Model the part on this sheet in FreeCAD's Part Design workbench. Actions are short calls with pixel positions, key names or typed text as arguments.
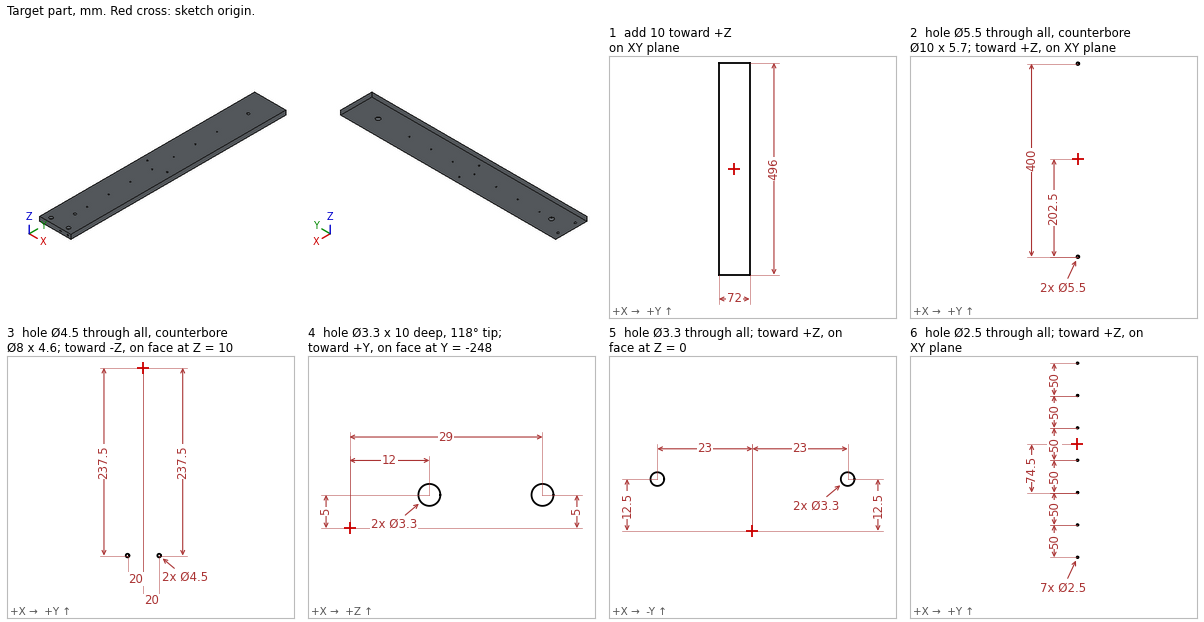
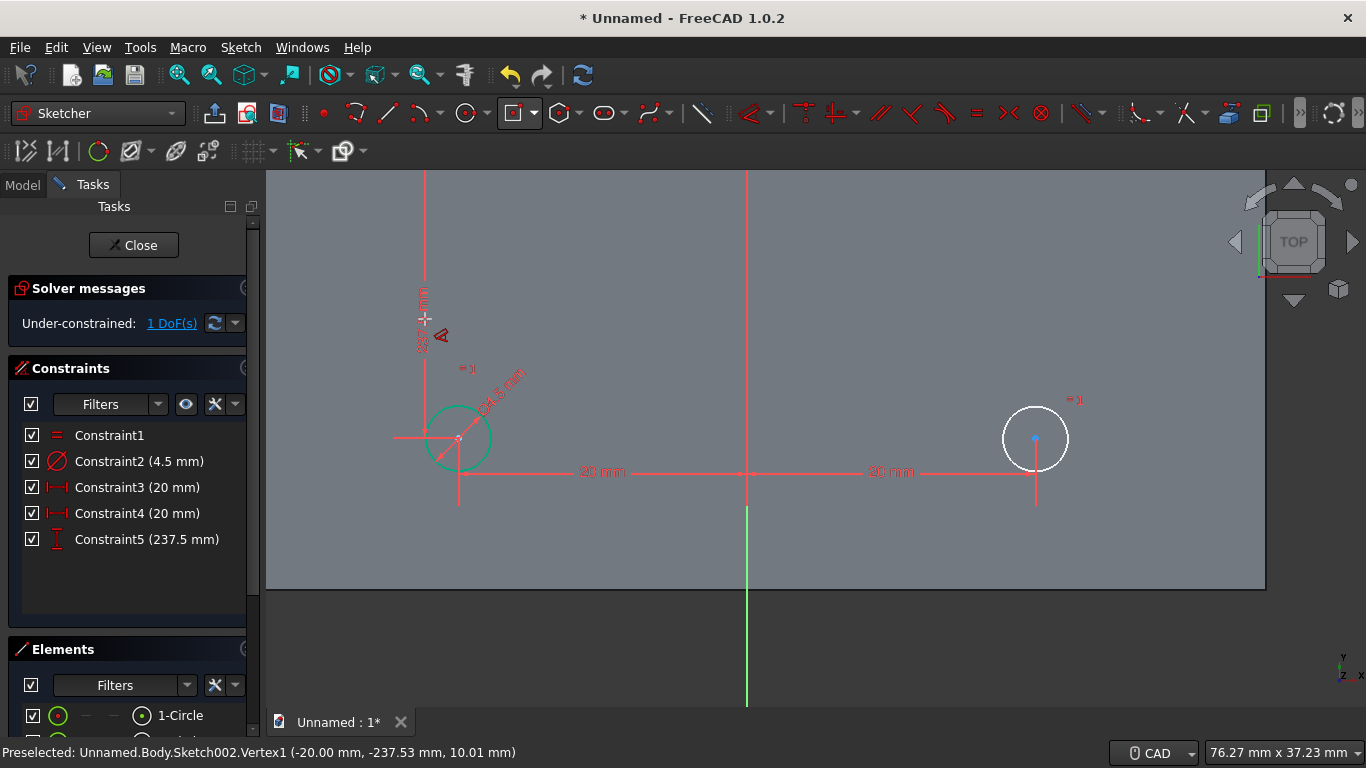
click(1036, 439)
click(1070, 319)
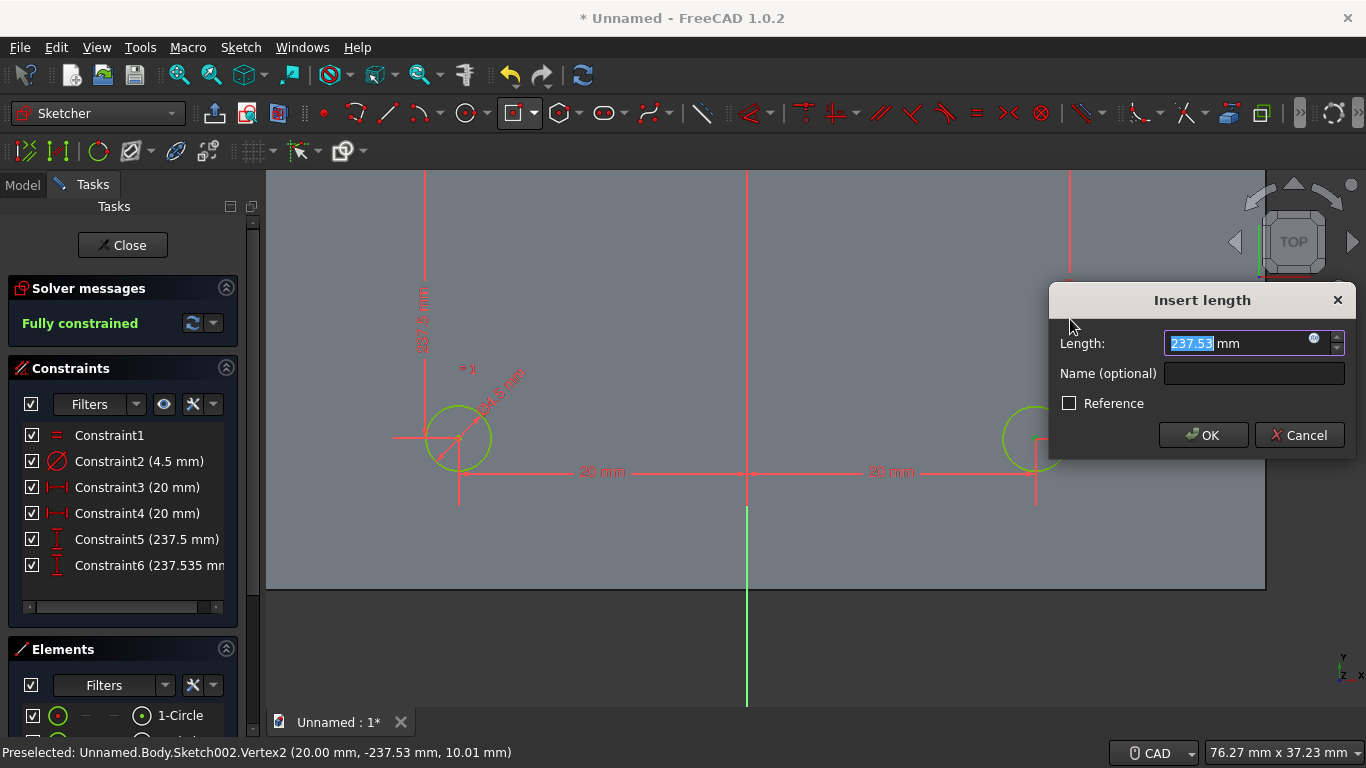
text(237.5)
key(Return)
key(Escape)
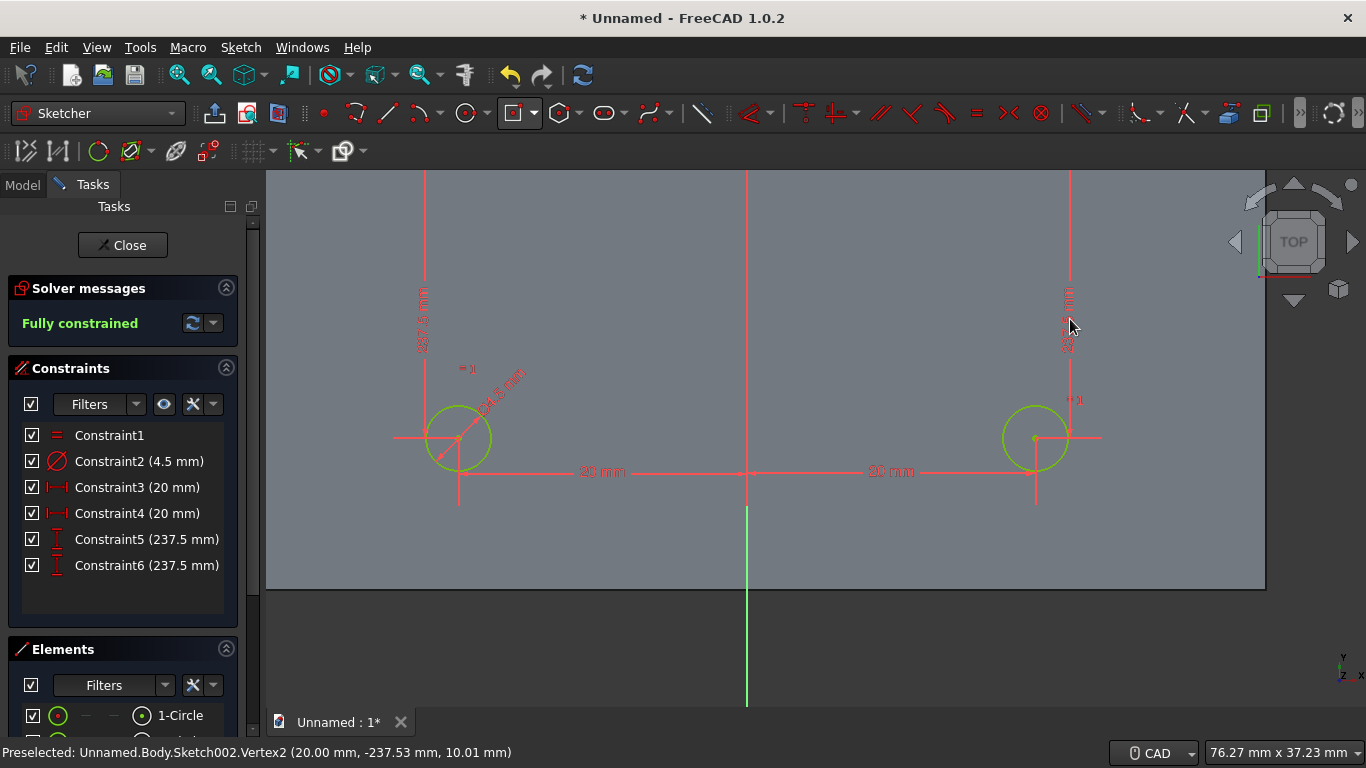
click(123, 245)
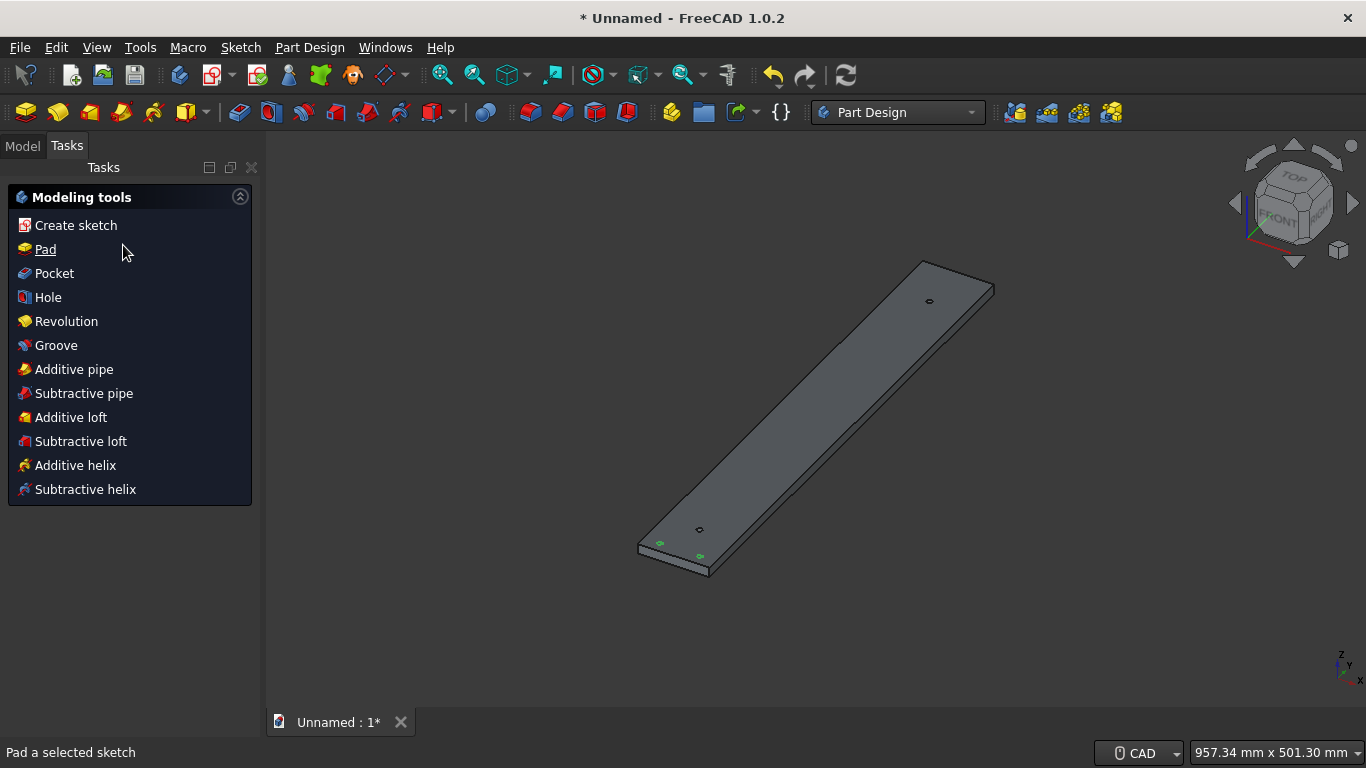
click(272, 112)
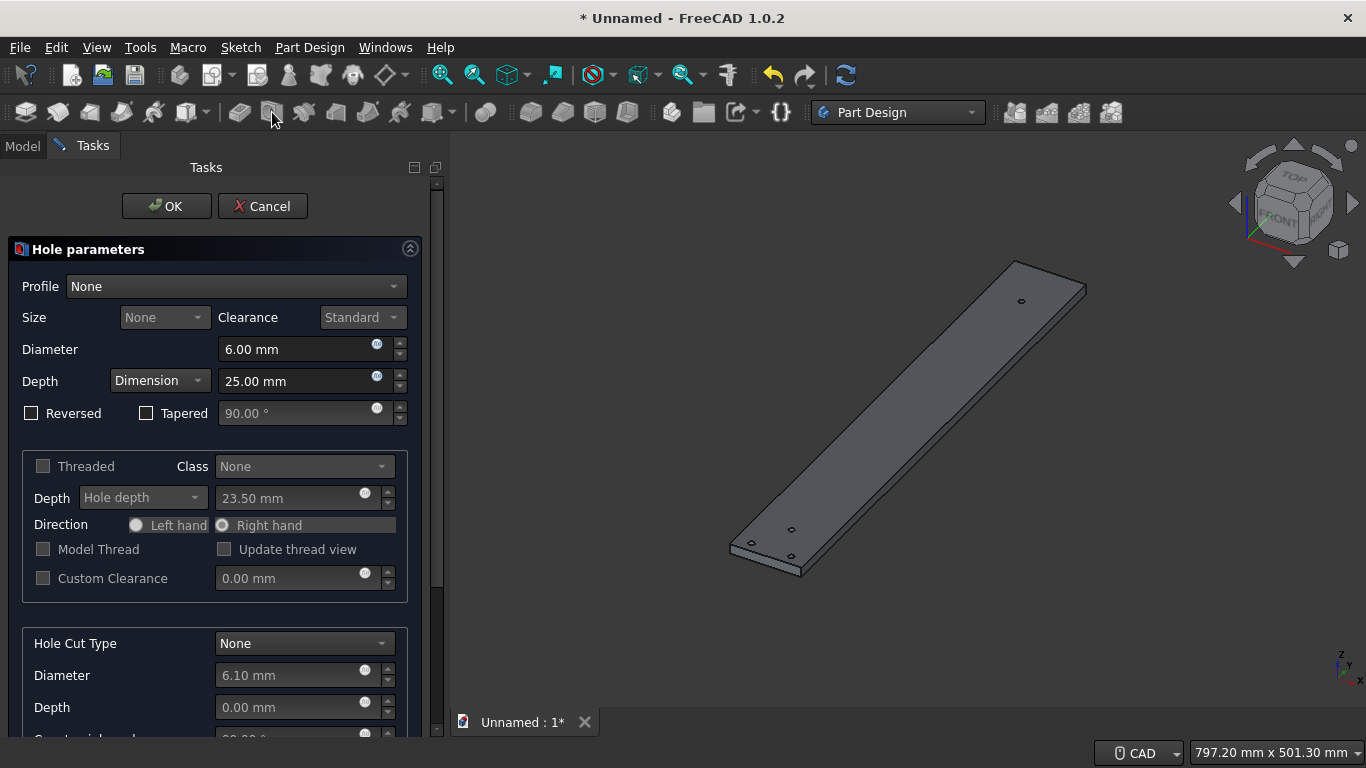
triple_click(305, 349)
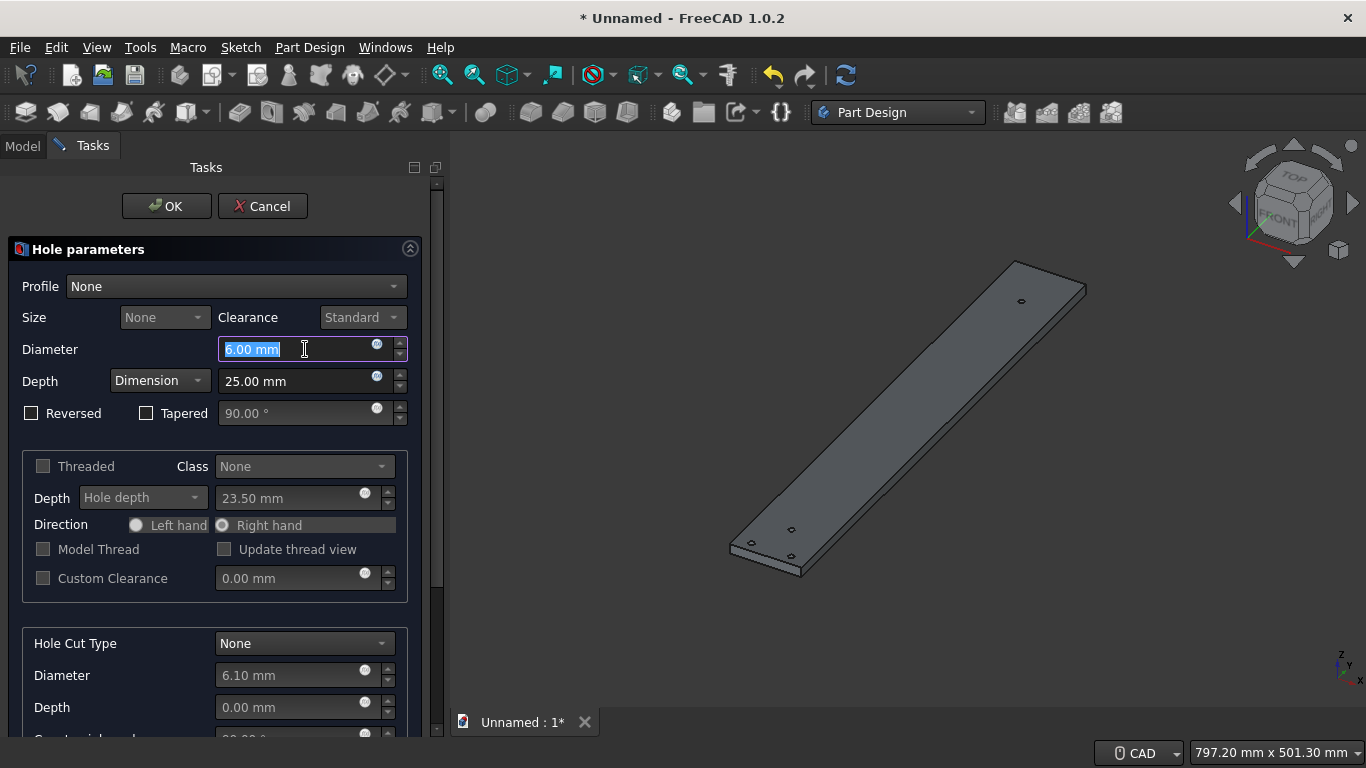
text(4.5)
key(Tab)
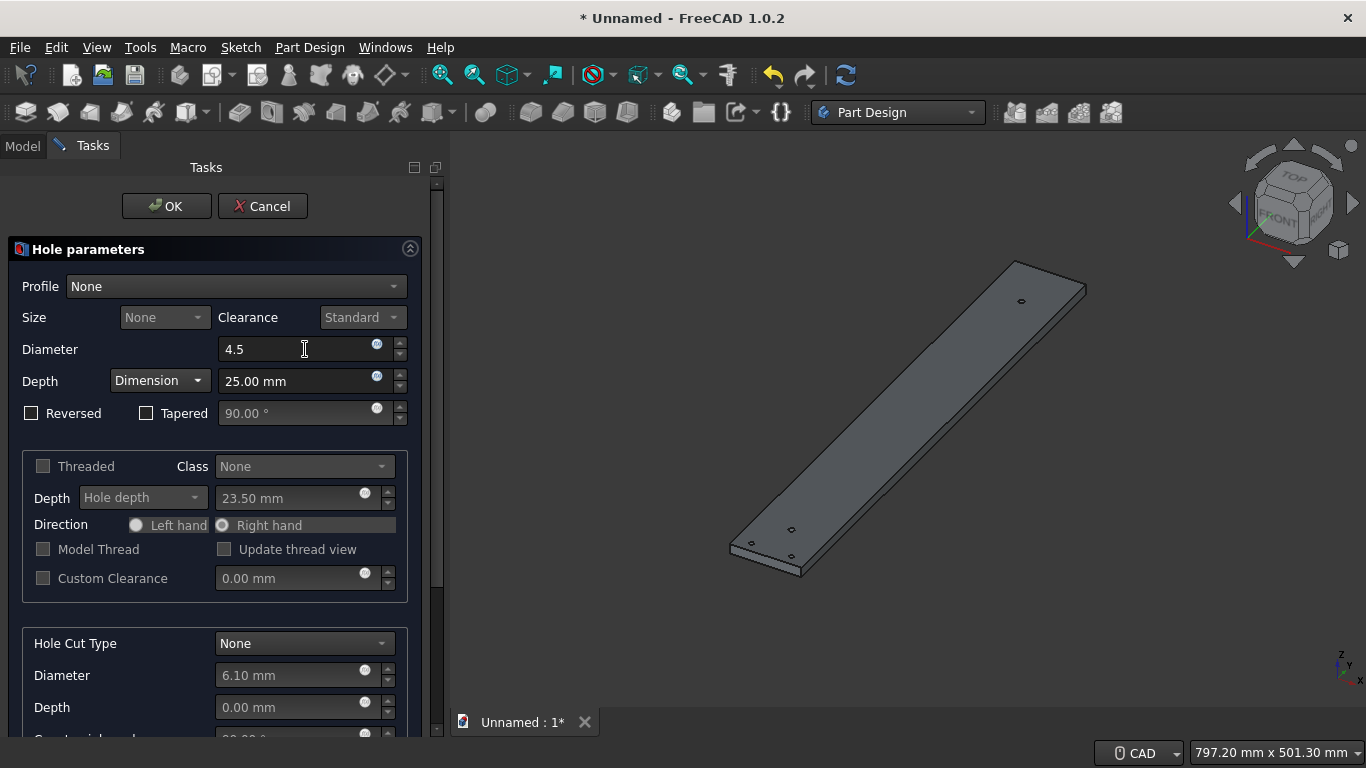
click(161, 380)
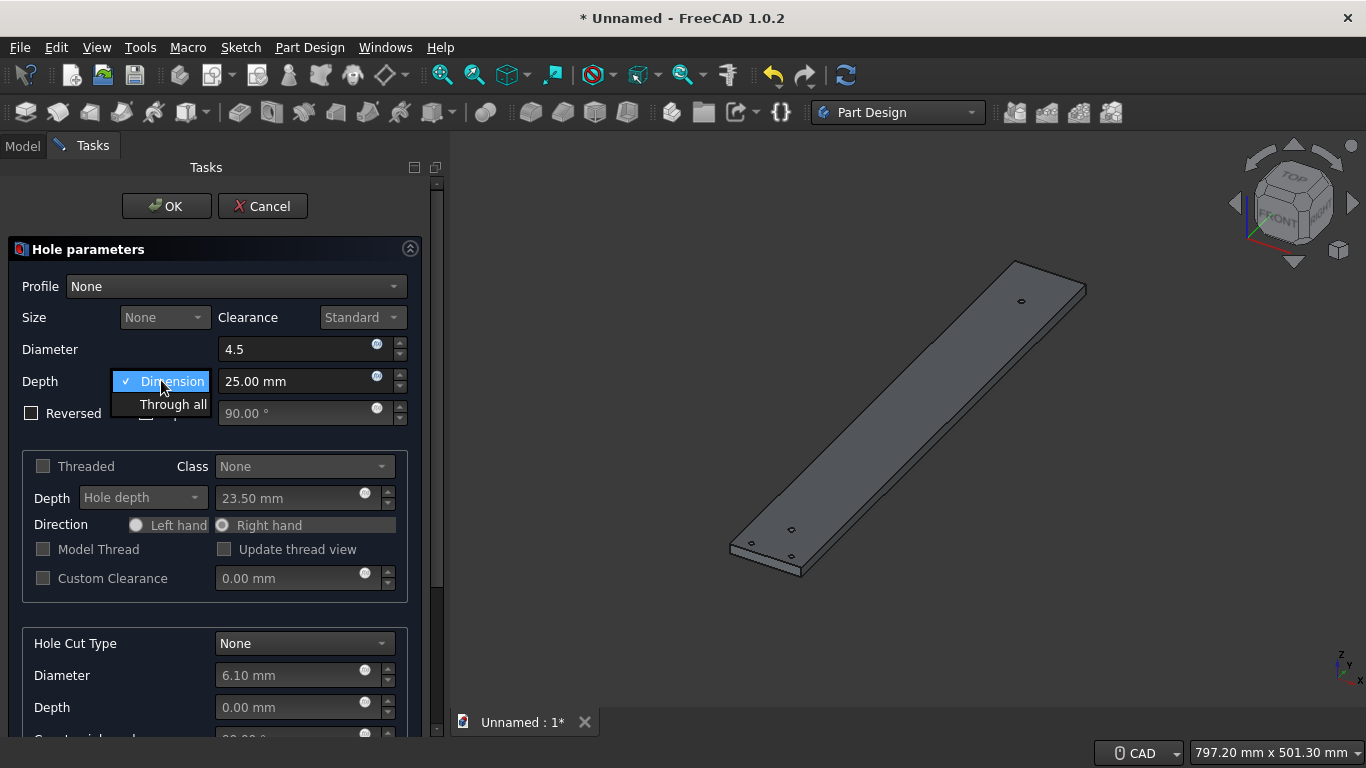
click(160, 404)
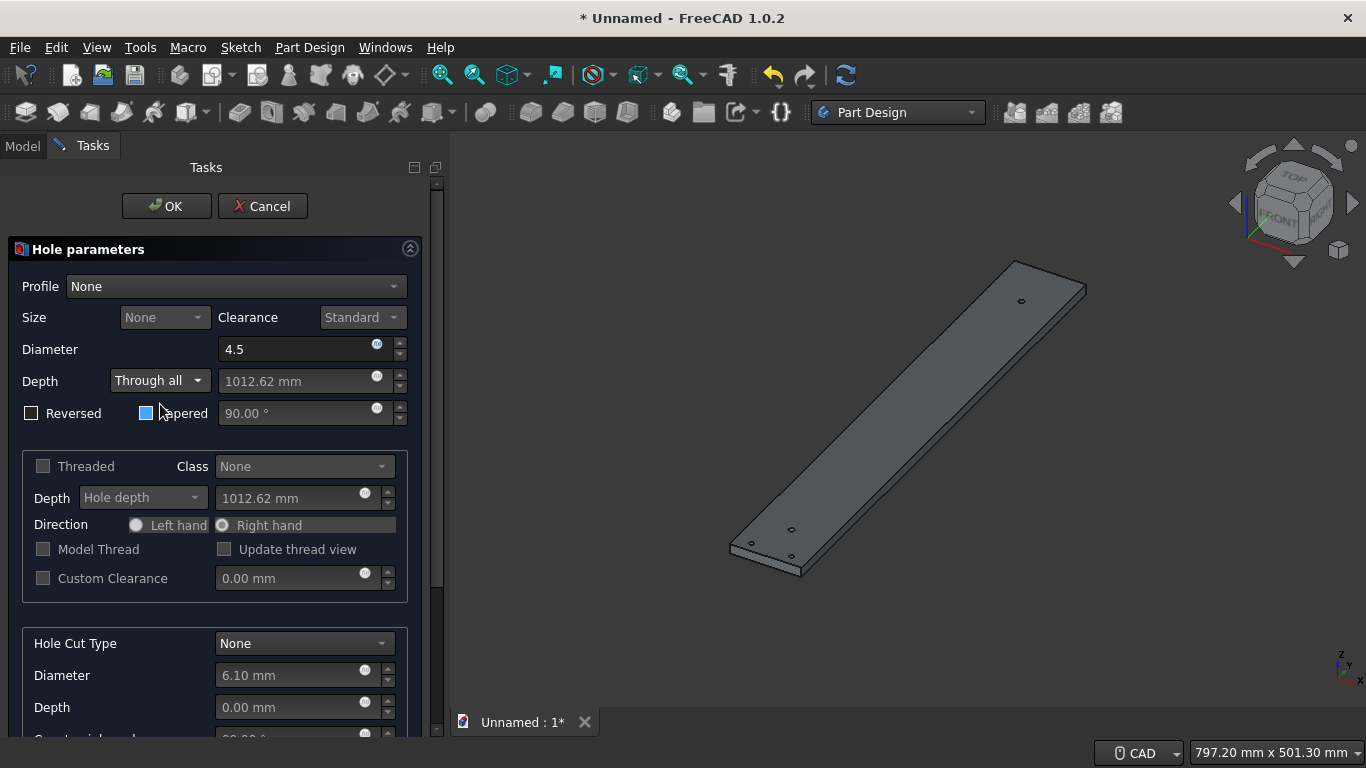
click(306, 644)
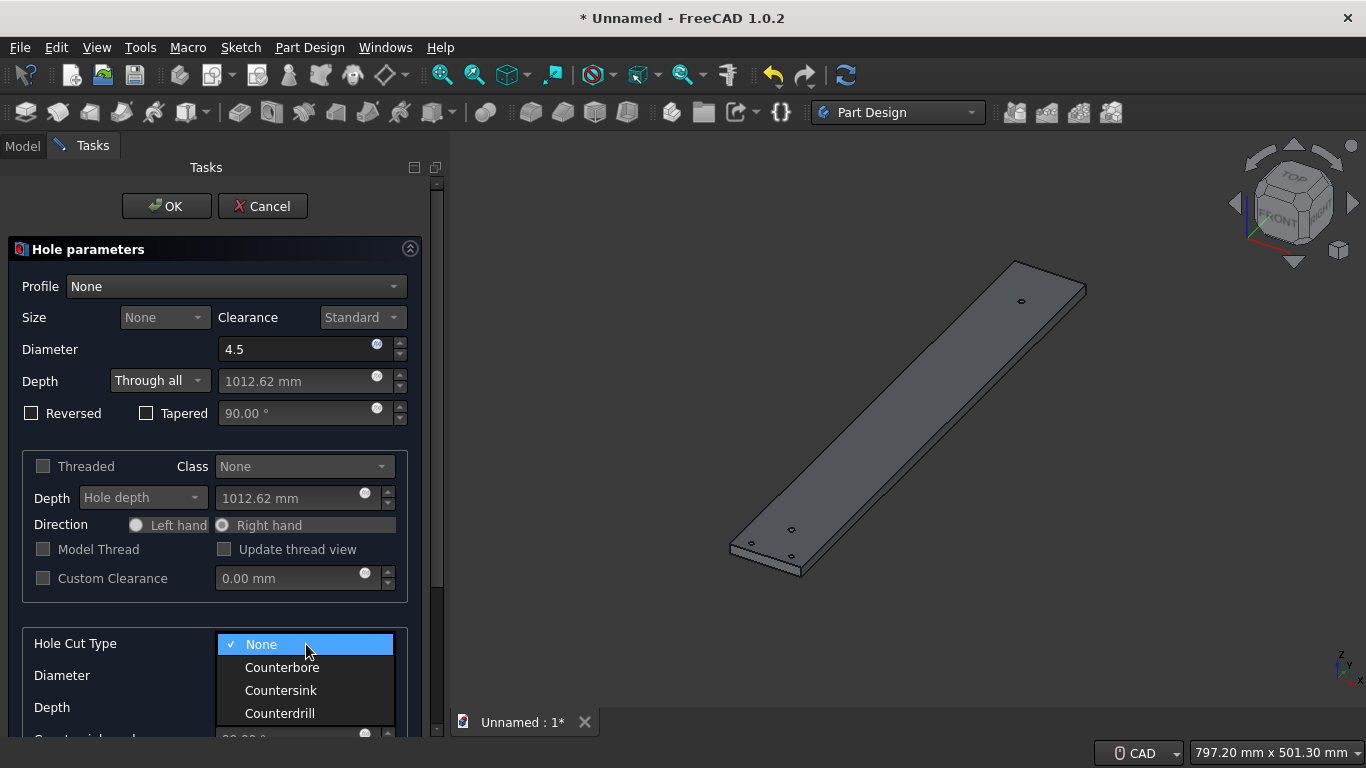
click(304, 668)